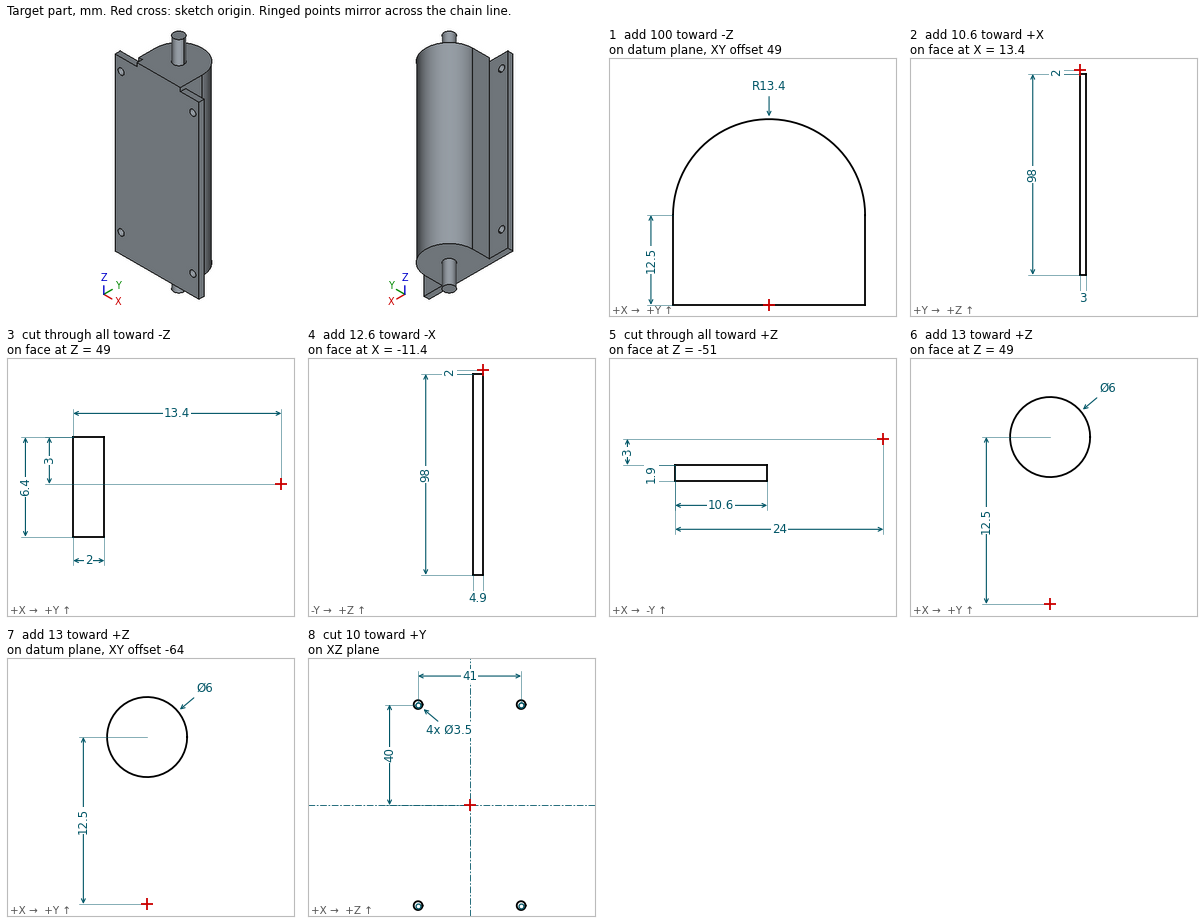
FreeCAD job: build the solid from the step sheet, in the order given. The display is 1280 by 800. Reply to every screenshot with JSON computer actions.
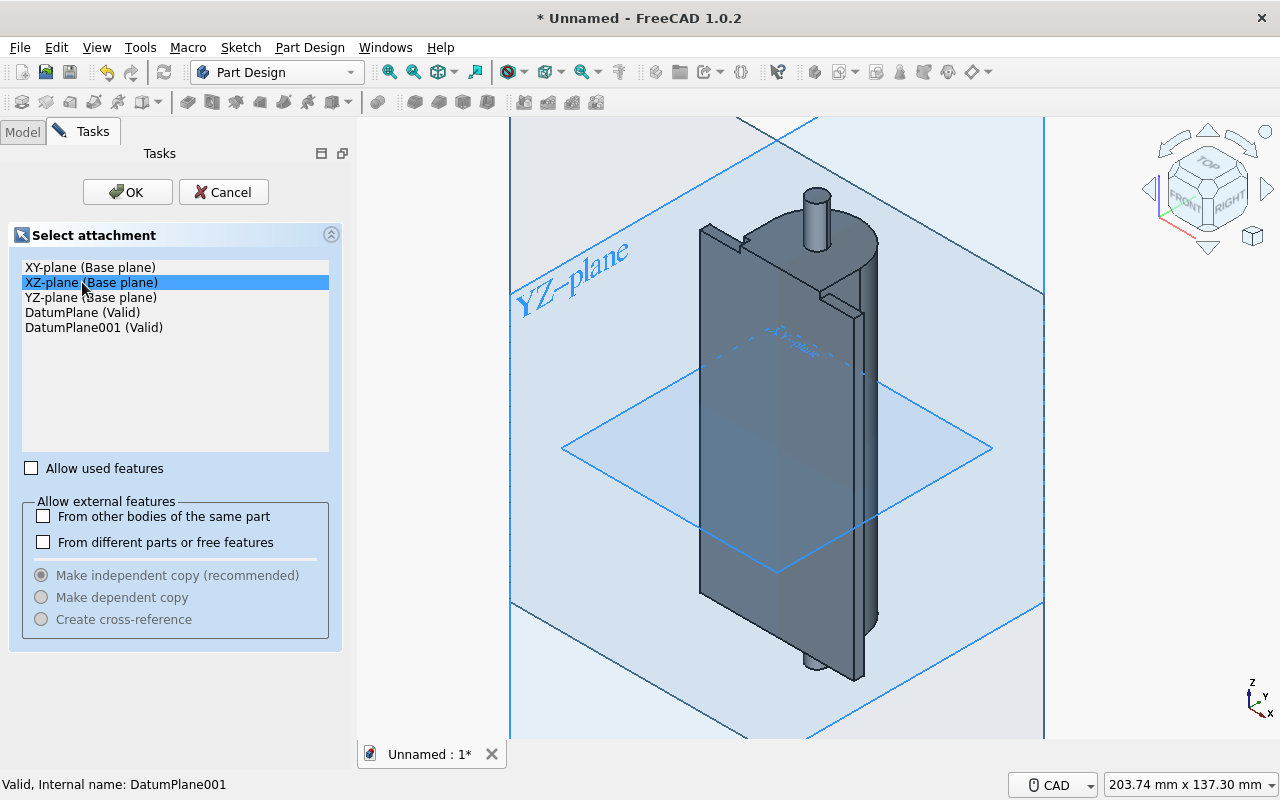
{"action": "left_click", "coordinate": [128, 192]}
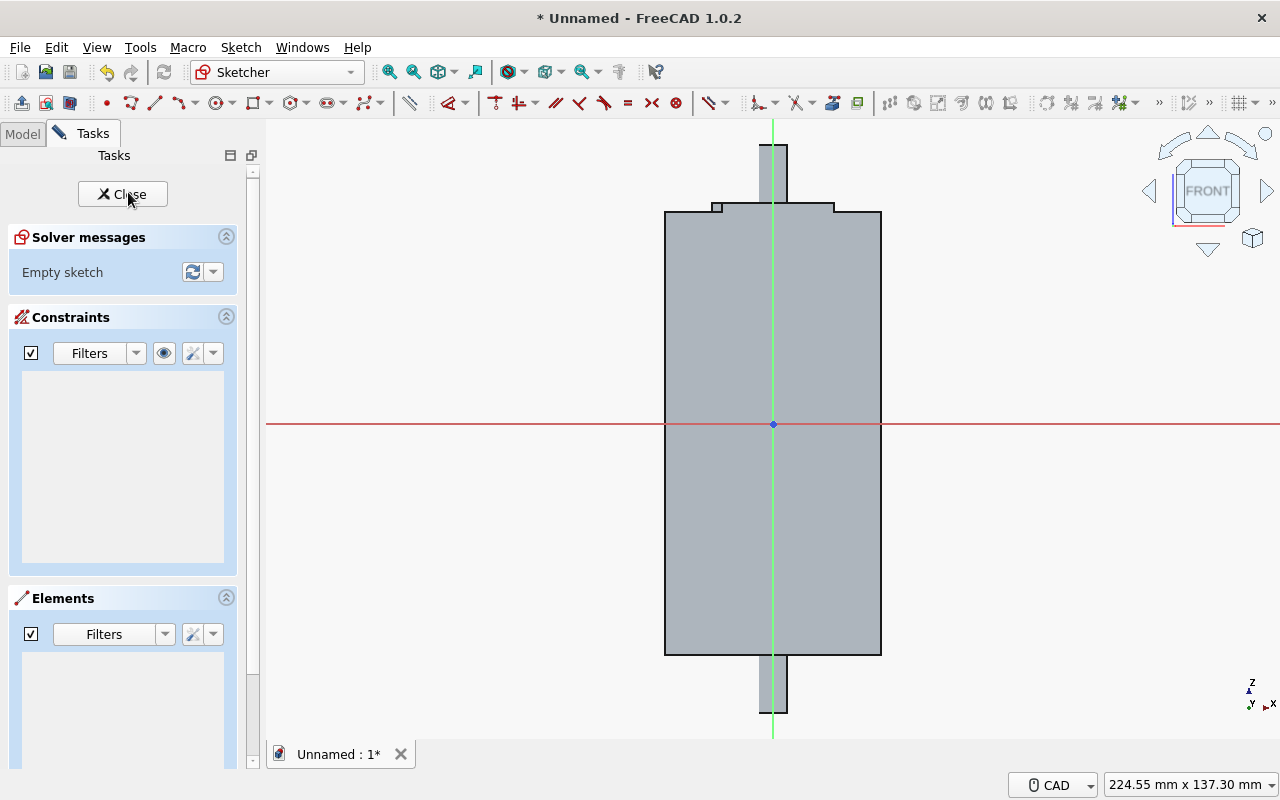
{"action": "left_click", "coordinate": [216, 104]}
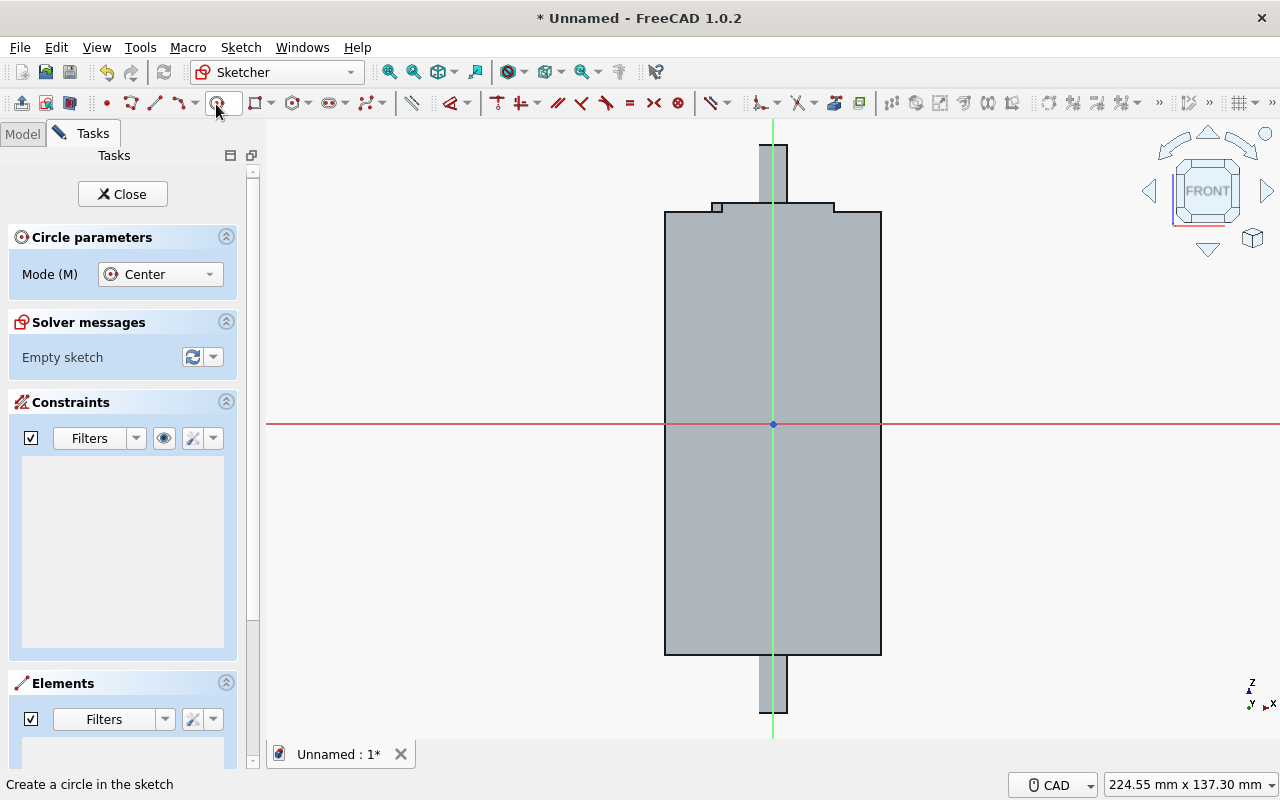
{"action": "scroll", "coordinate": [680, 244], "scroll_direction": "up", "scroll_amount": 6}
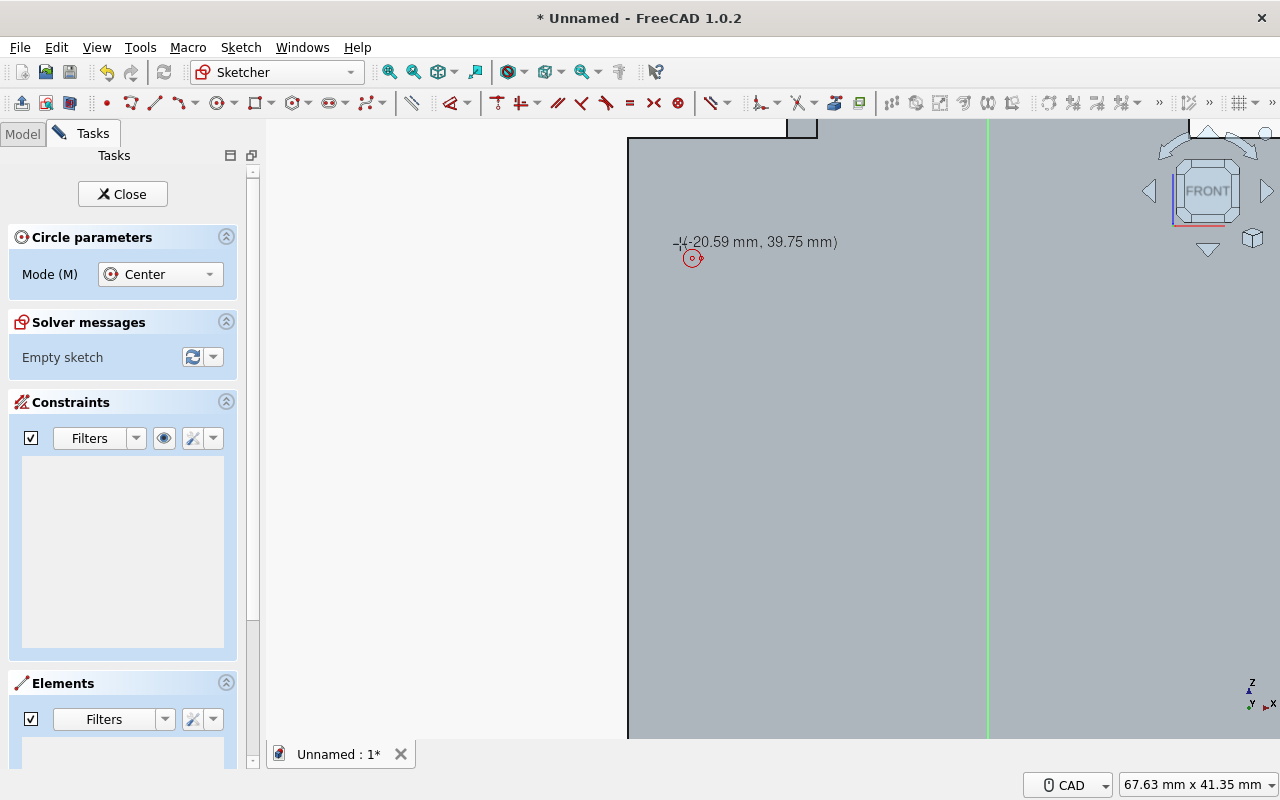
{"action": "left_click", "coordinate": [680, 243]}
{"action": "left_click", "coordinate": [699, 224]}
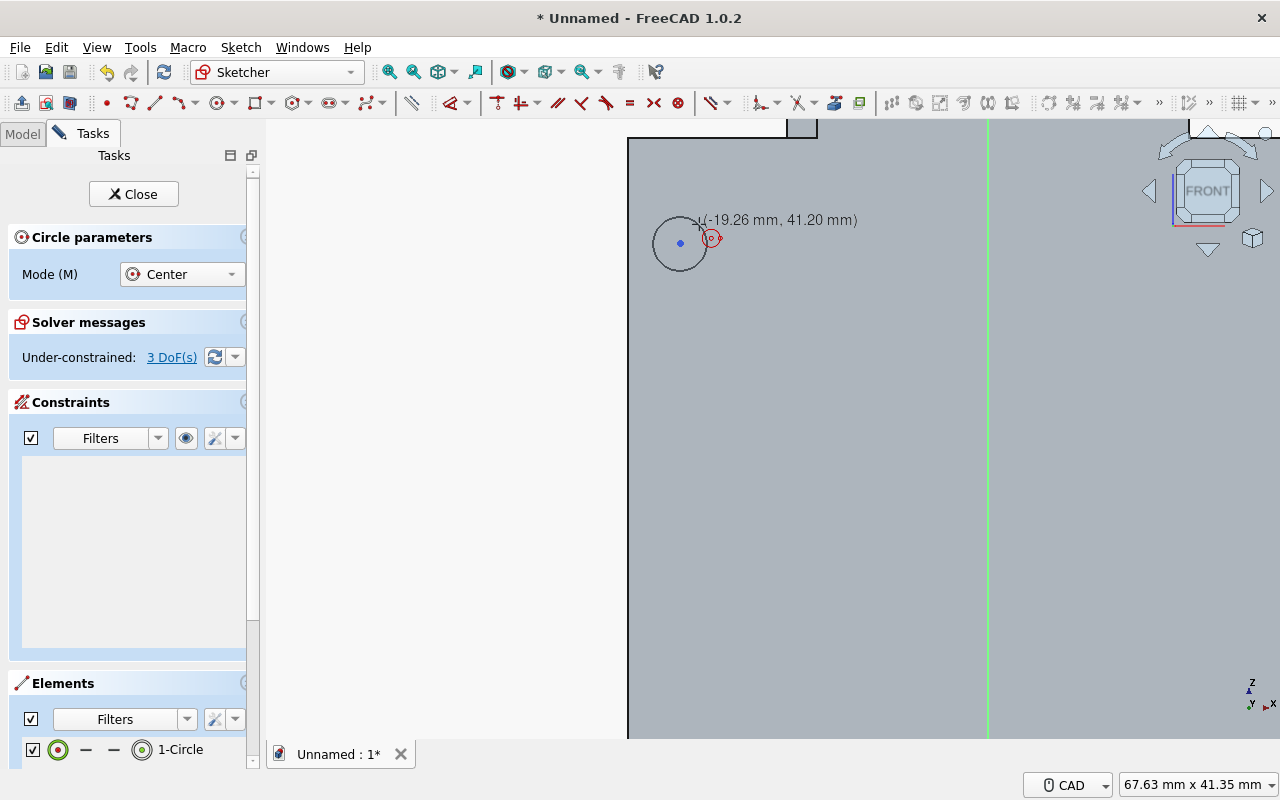
{"action": "scroll", "coordinate": [582, 251], "scroll_direction": "down", "scroll_amount": 6}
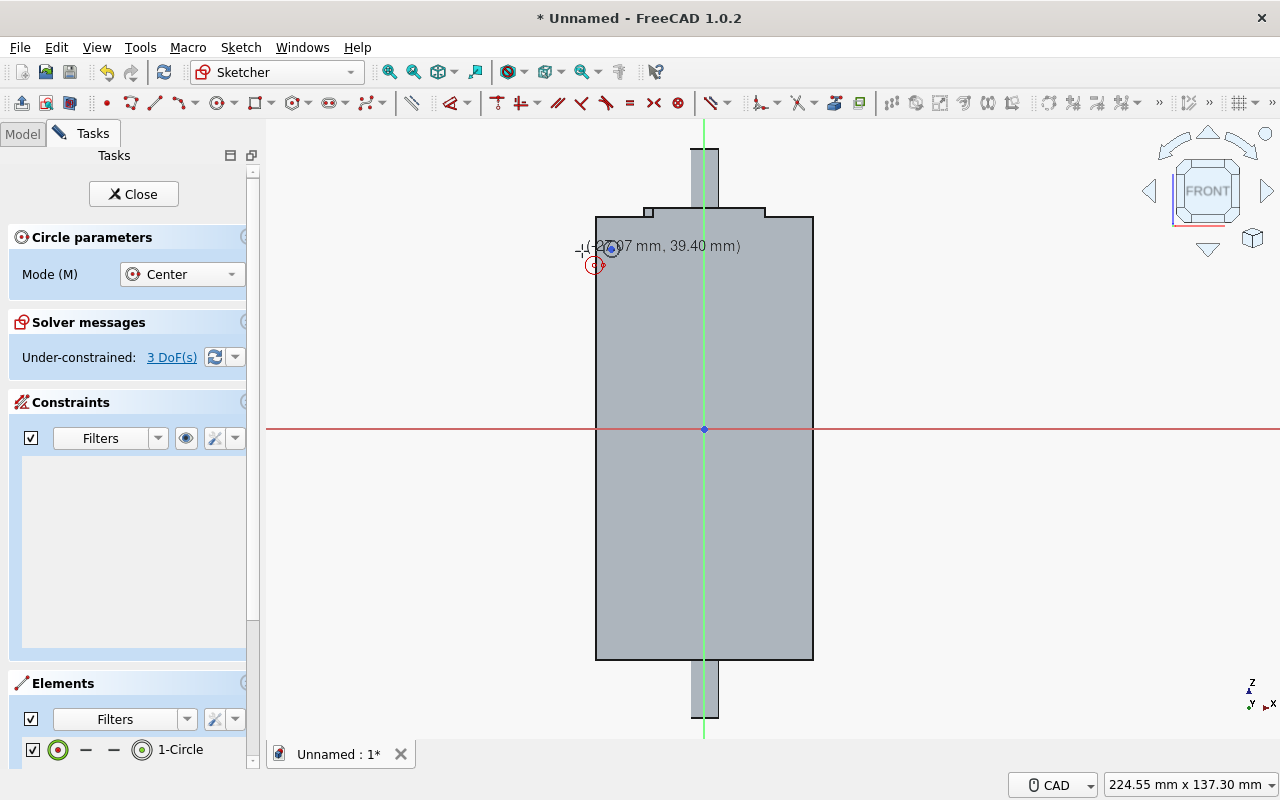
{"action": "scroll", "coordinate": [797, 249], "scroll_direction": "up", "scroll_amount": 6}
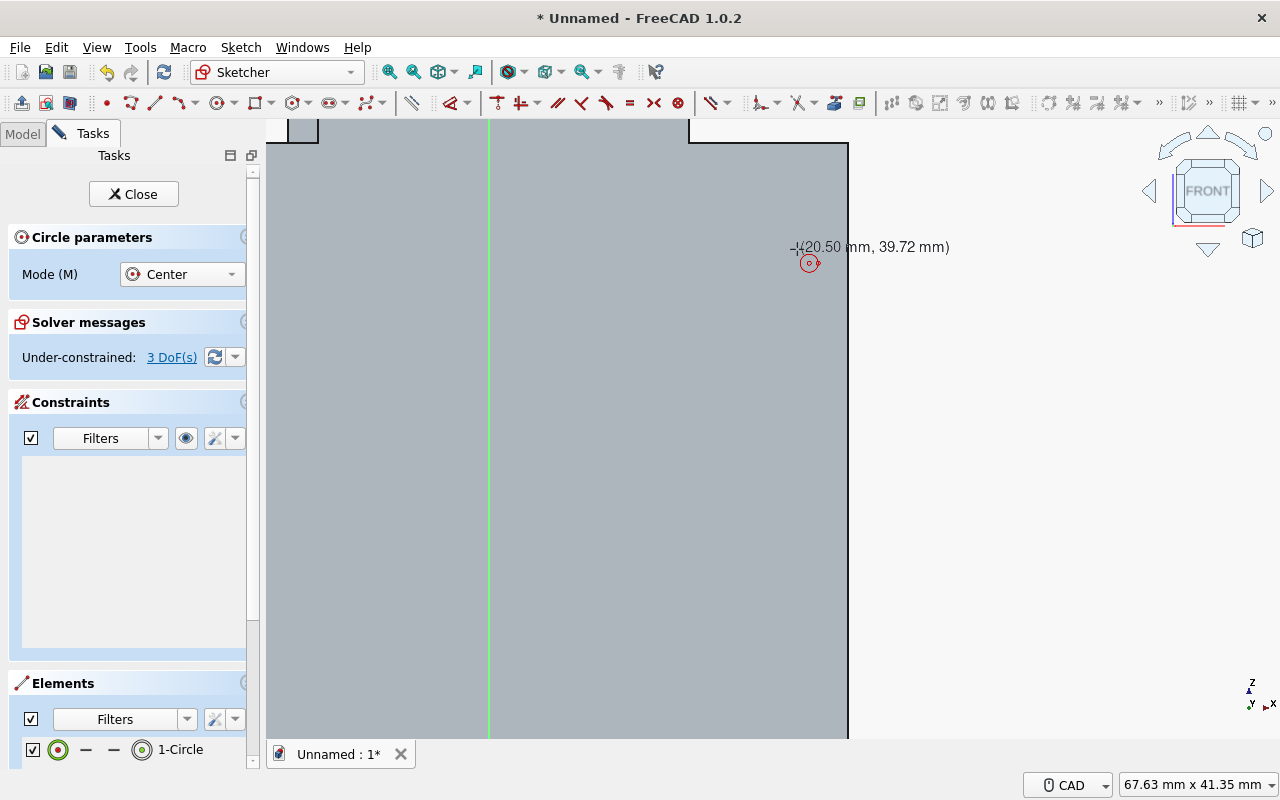
{"action": "left_click", "coordinate": [796, 248]}
{"action": "left_click", "coordinate": [814, 229]}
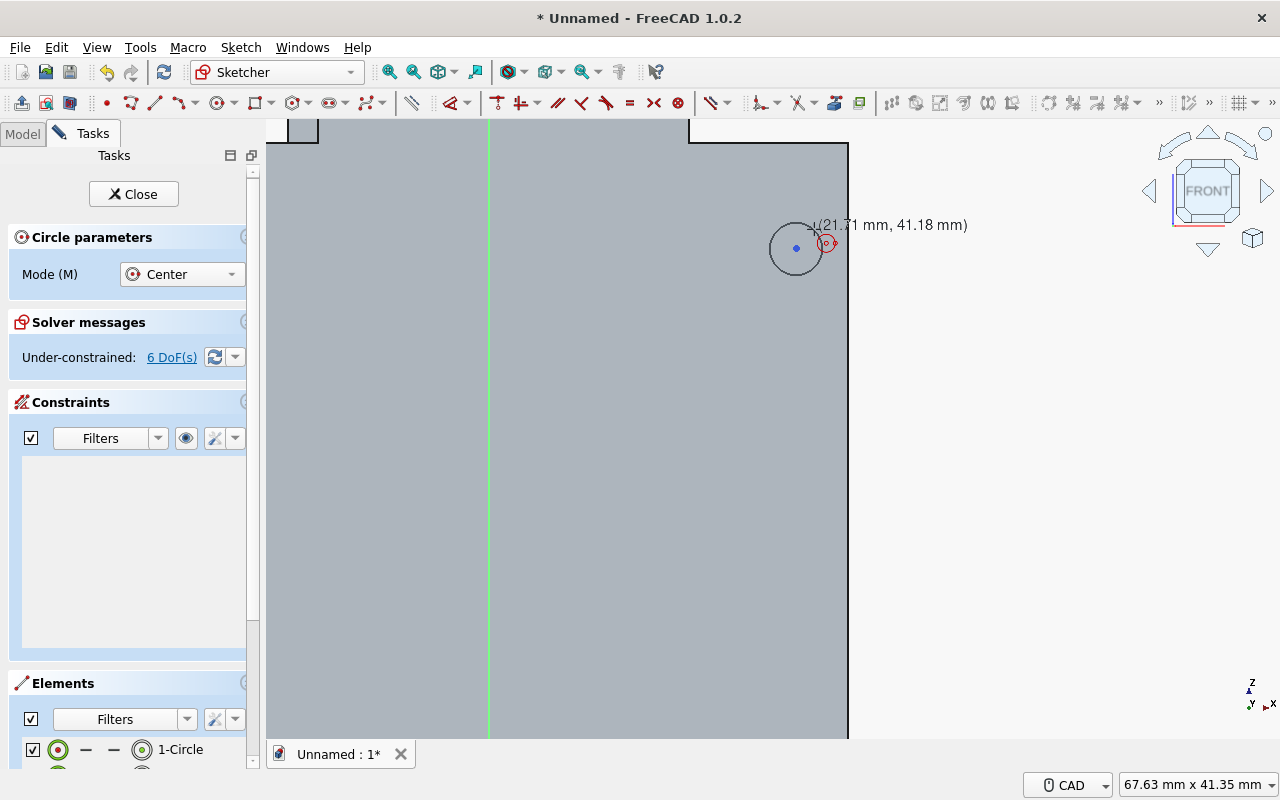
{"action": "scroll", "coordinate": [798, 249], "scroll_direction": "down", "scroll_amount": 6}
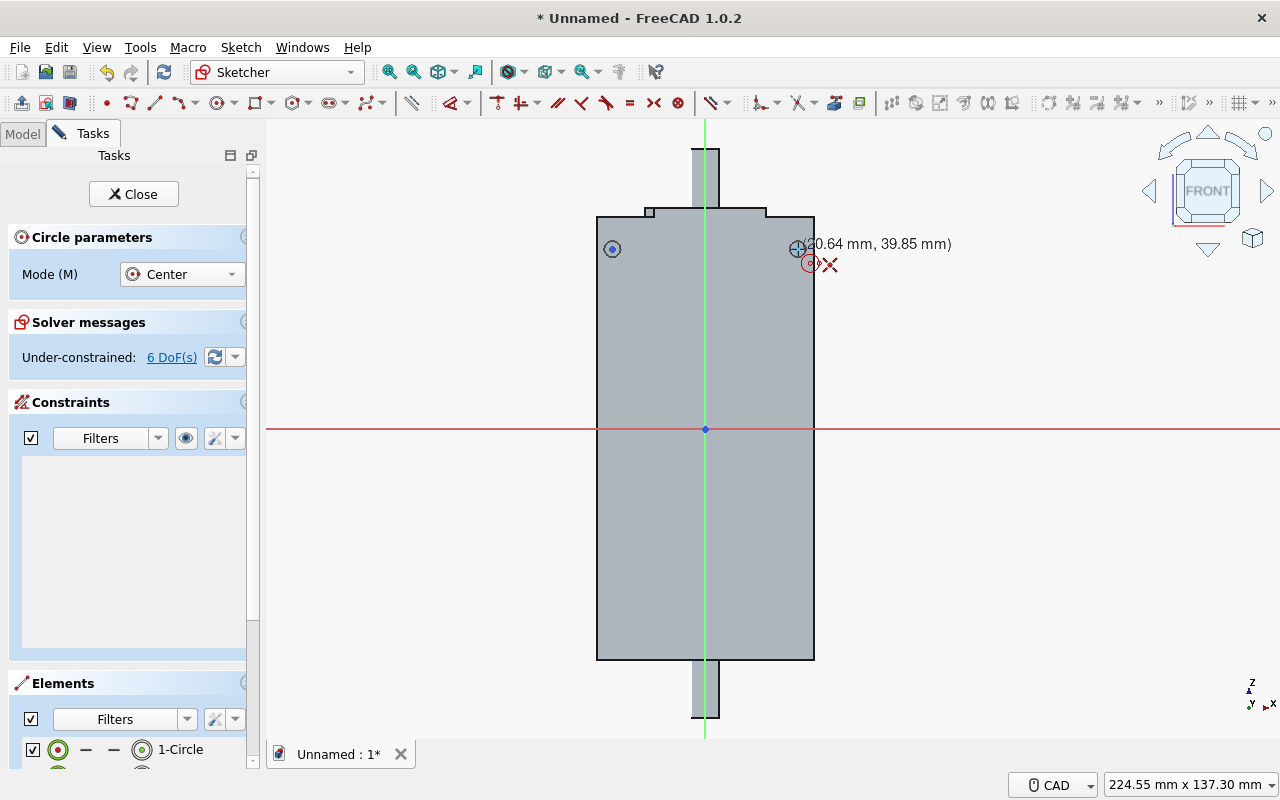
{"action": "scroll", "coordinate": [798, 610], "scroll_direction": "up", "scroll_amount": 6}